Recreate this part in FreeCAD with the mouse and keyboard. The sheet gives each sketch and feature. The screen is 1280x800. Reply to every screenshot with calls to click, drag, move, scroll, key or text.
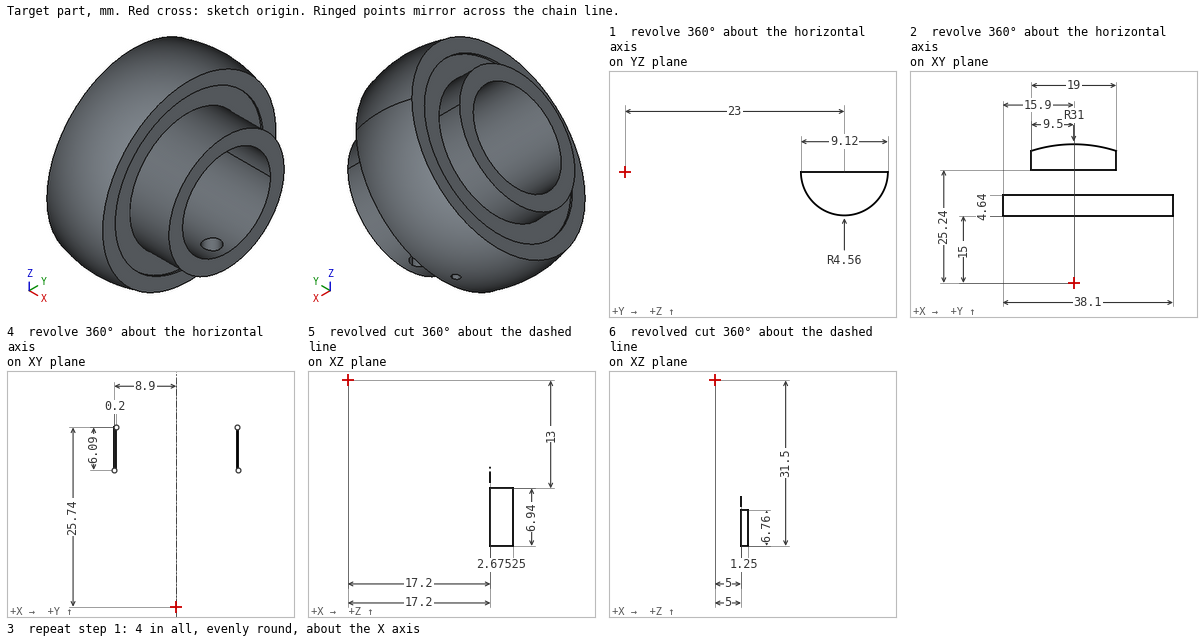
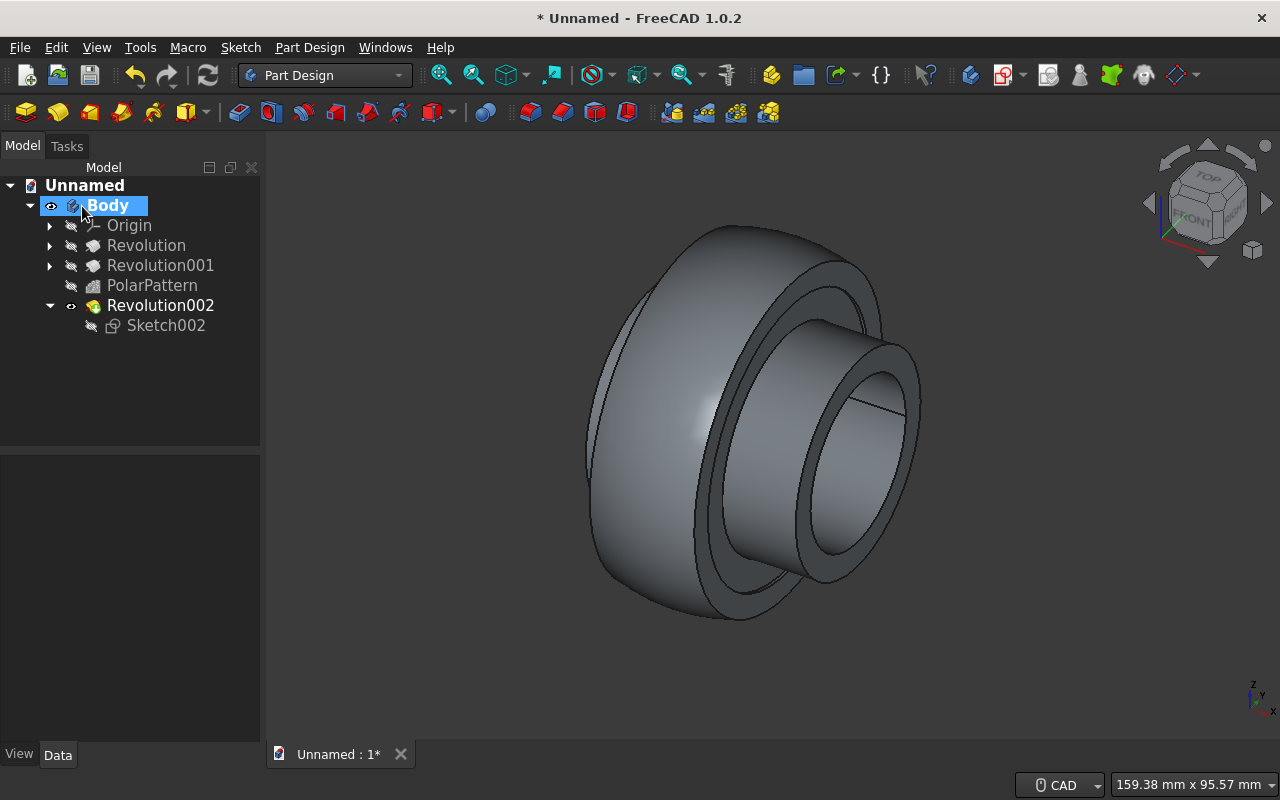
click(1004, 76)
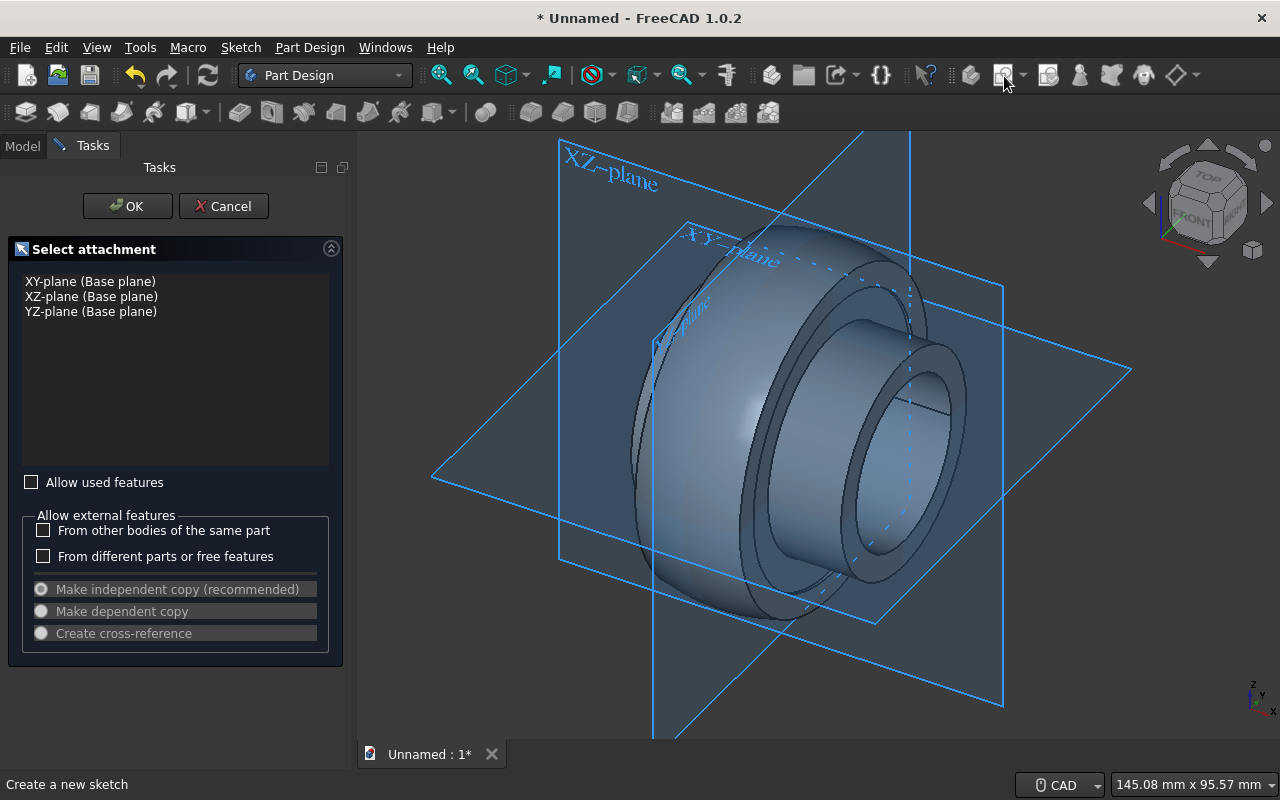
click(82, 296)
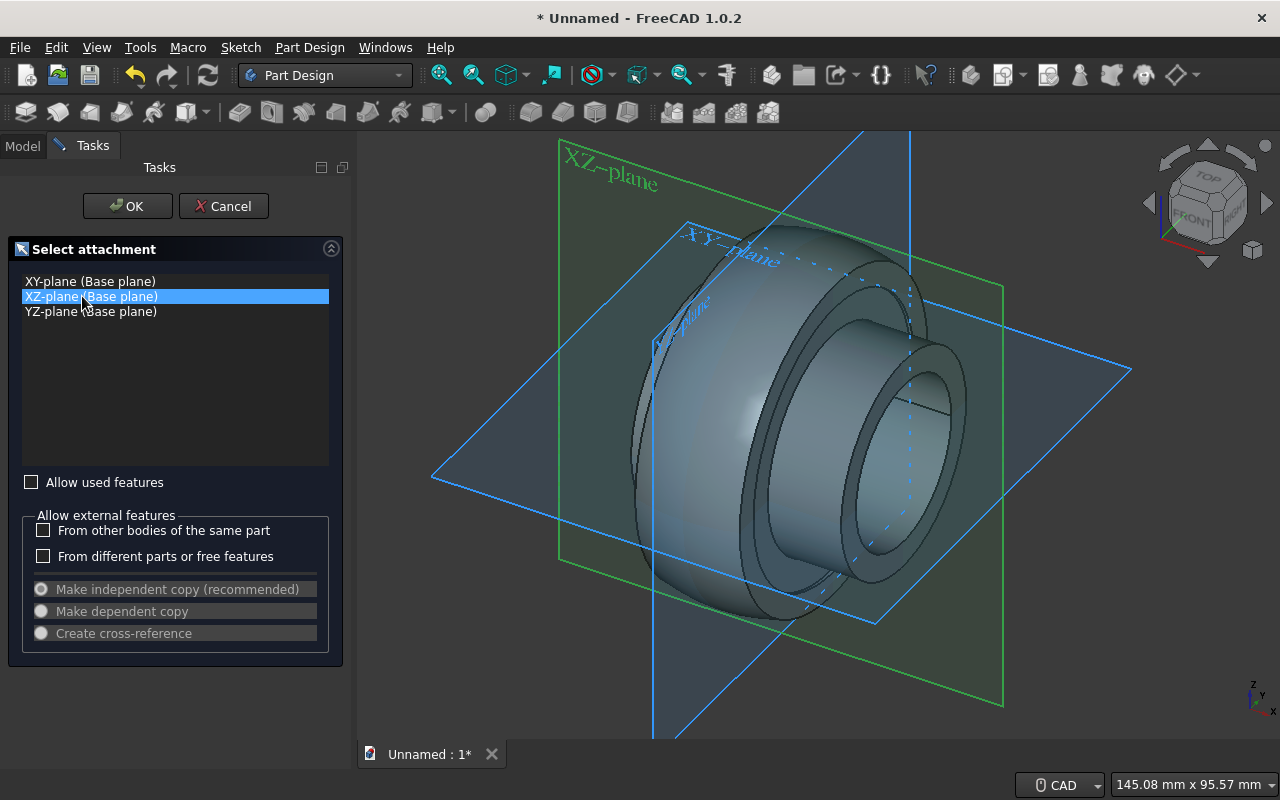
click(128, 206)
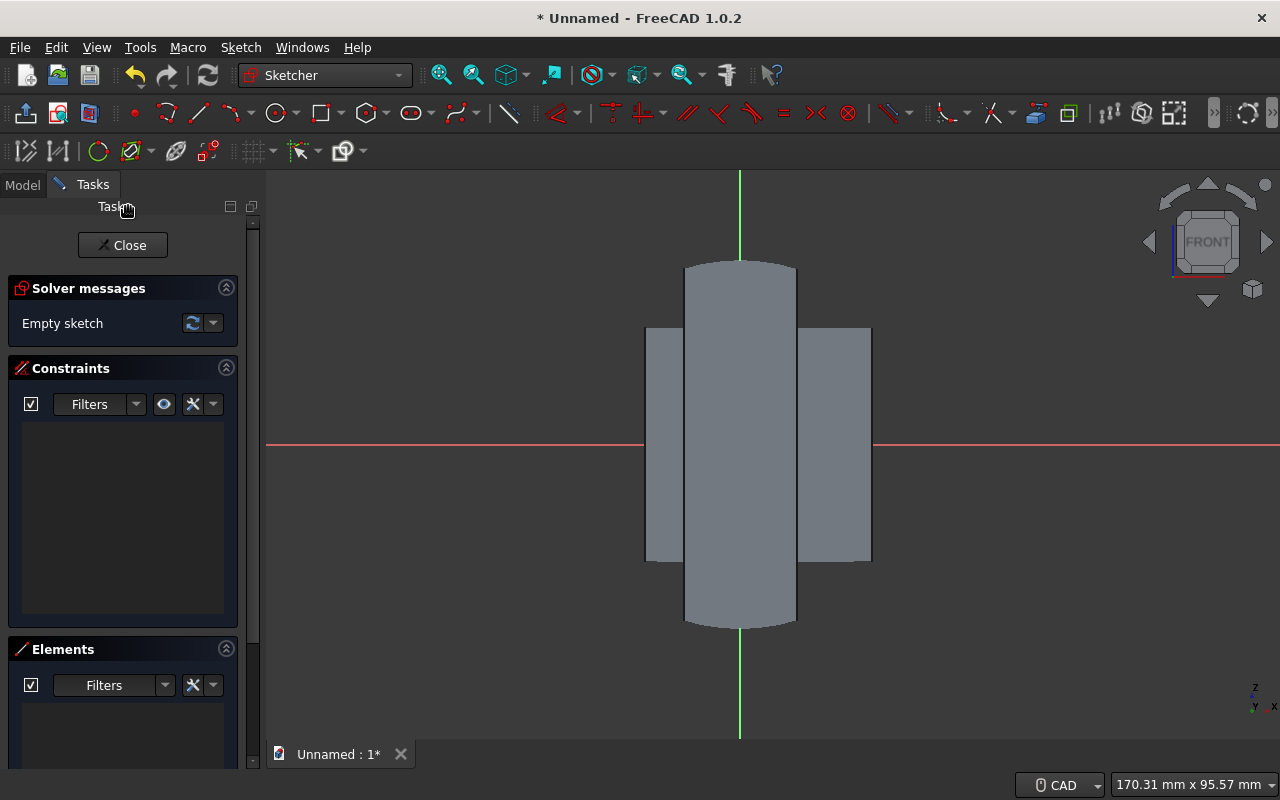
click(90, 114)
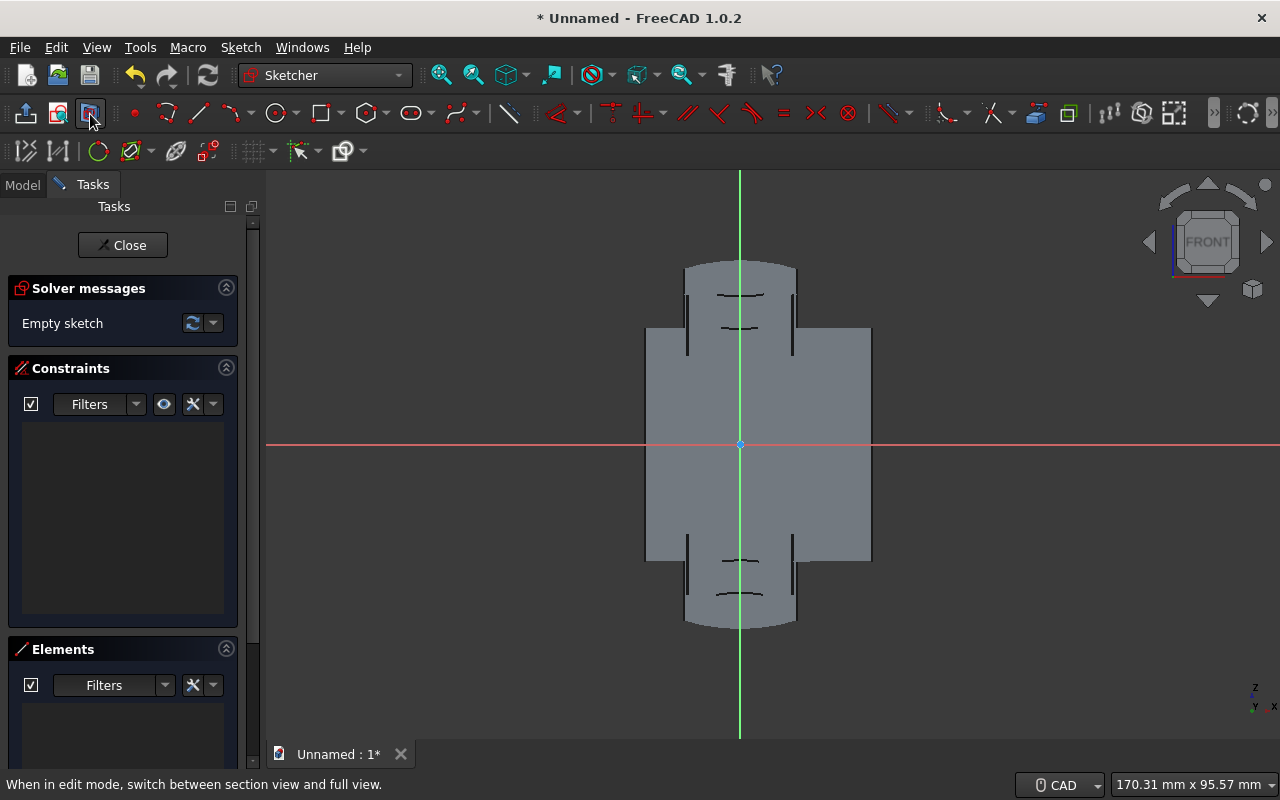
scroll(840, 525, up, 6)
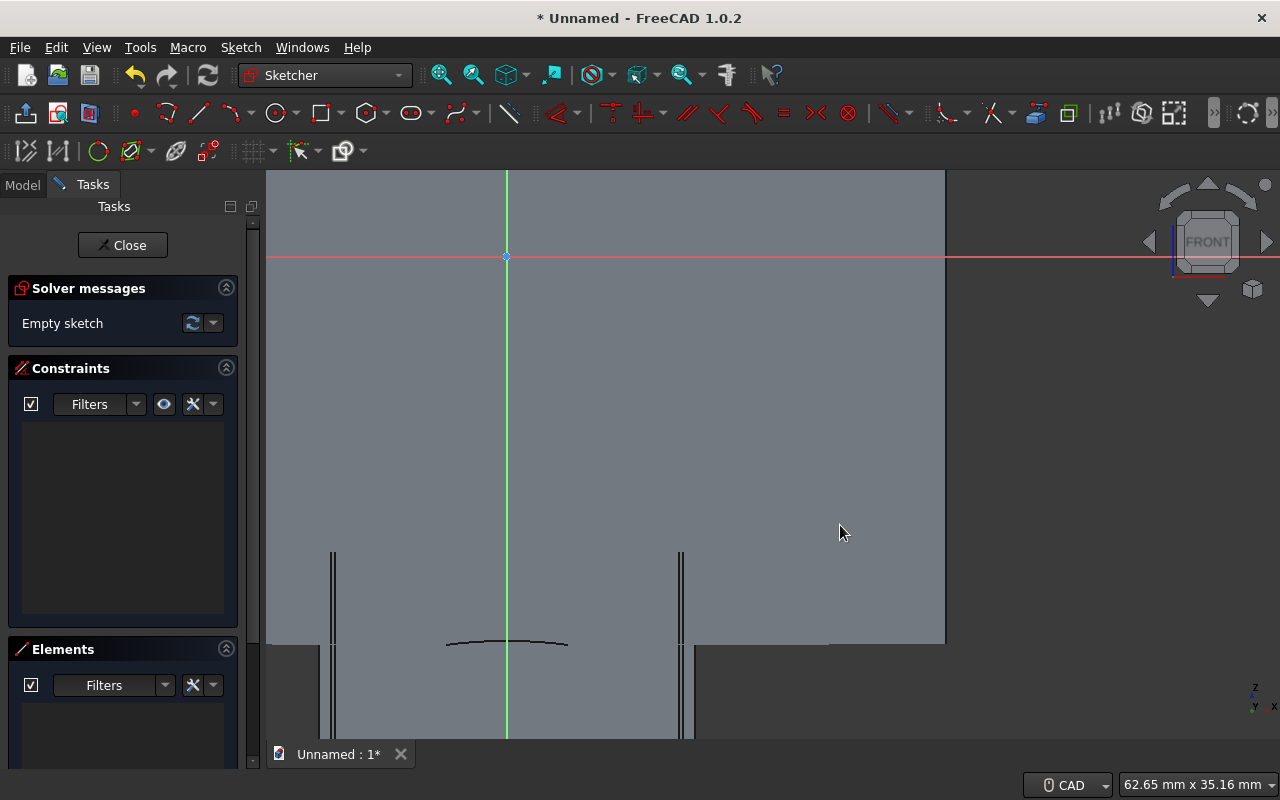
click(322, 114)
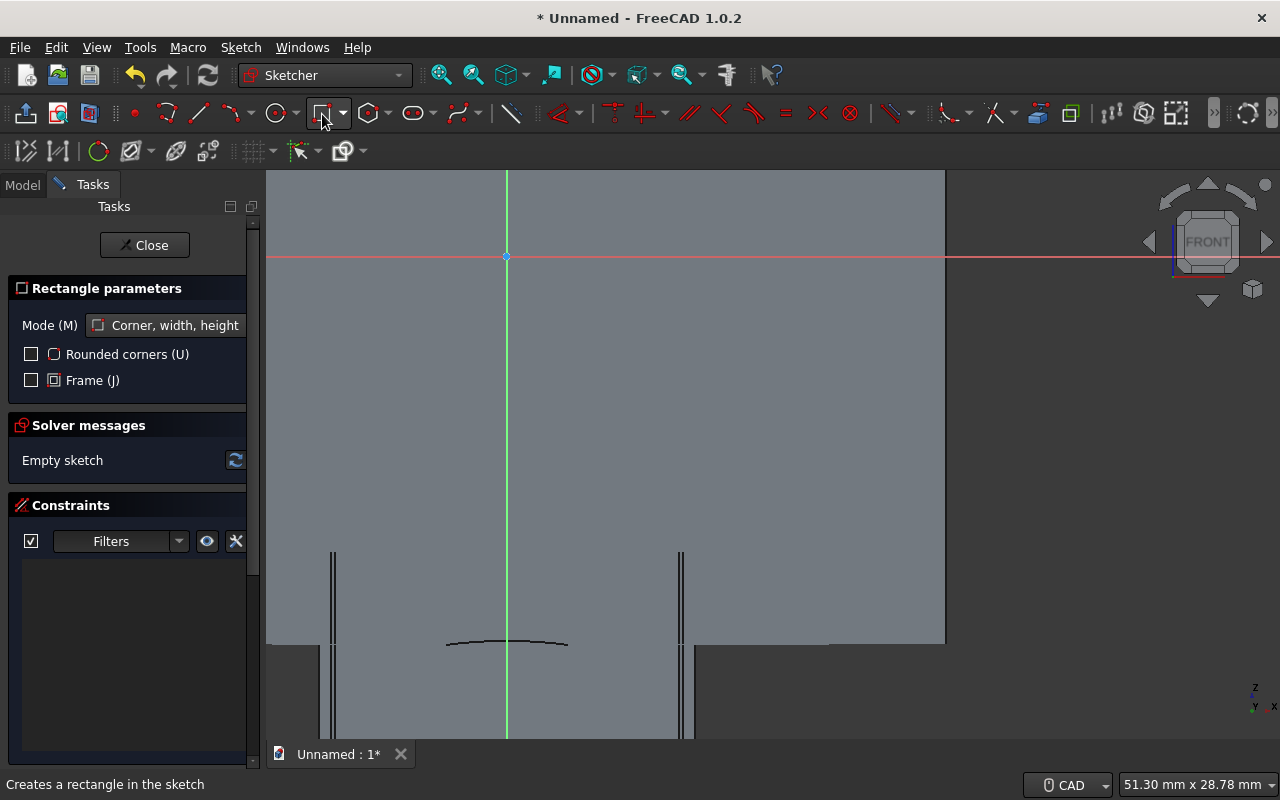
click(847, 514)
click(900, 651)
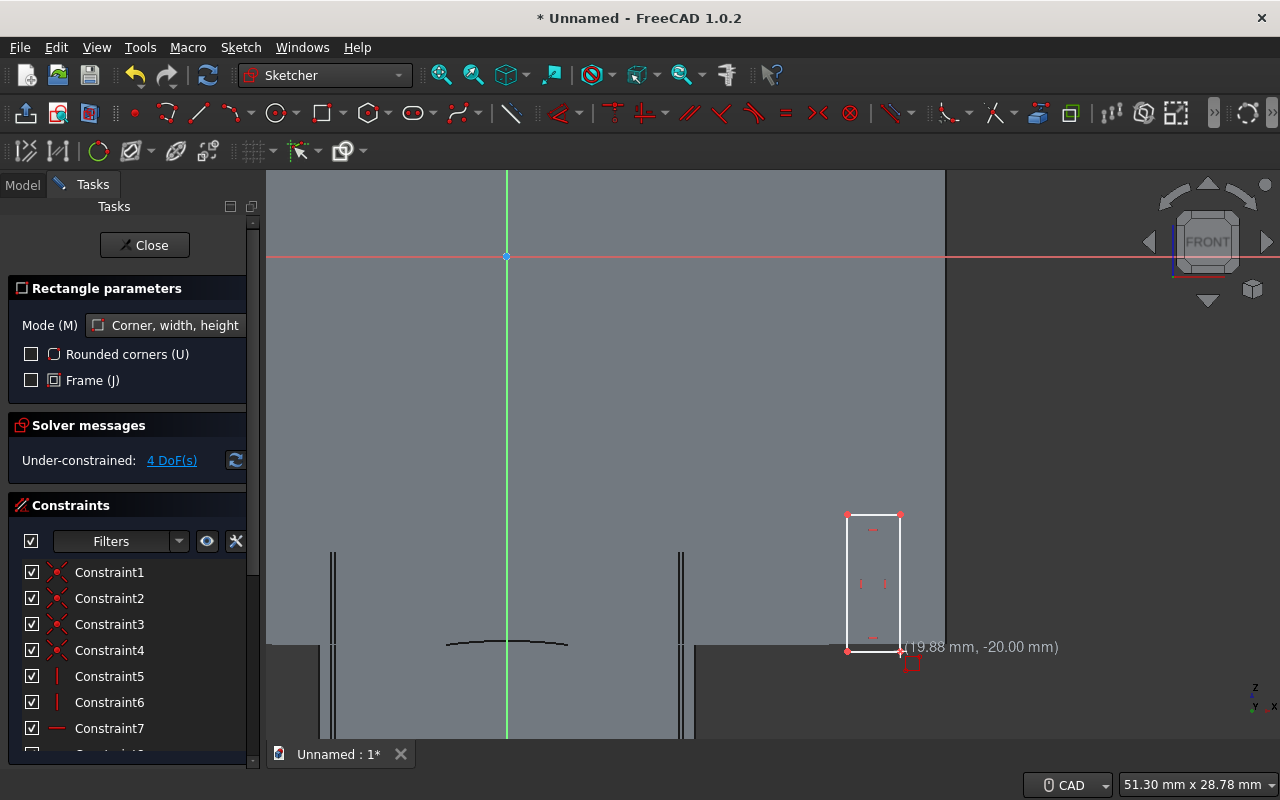
click(200, 114)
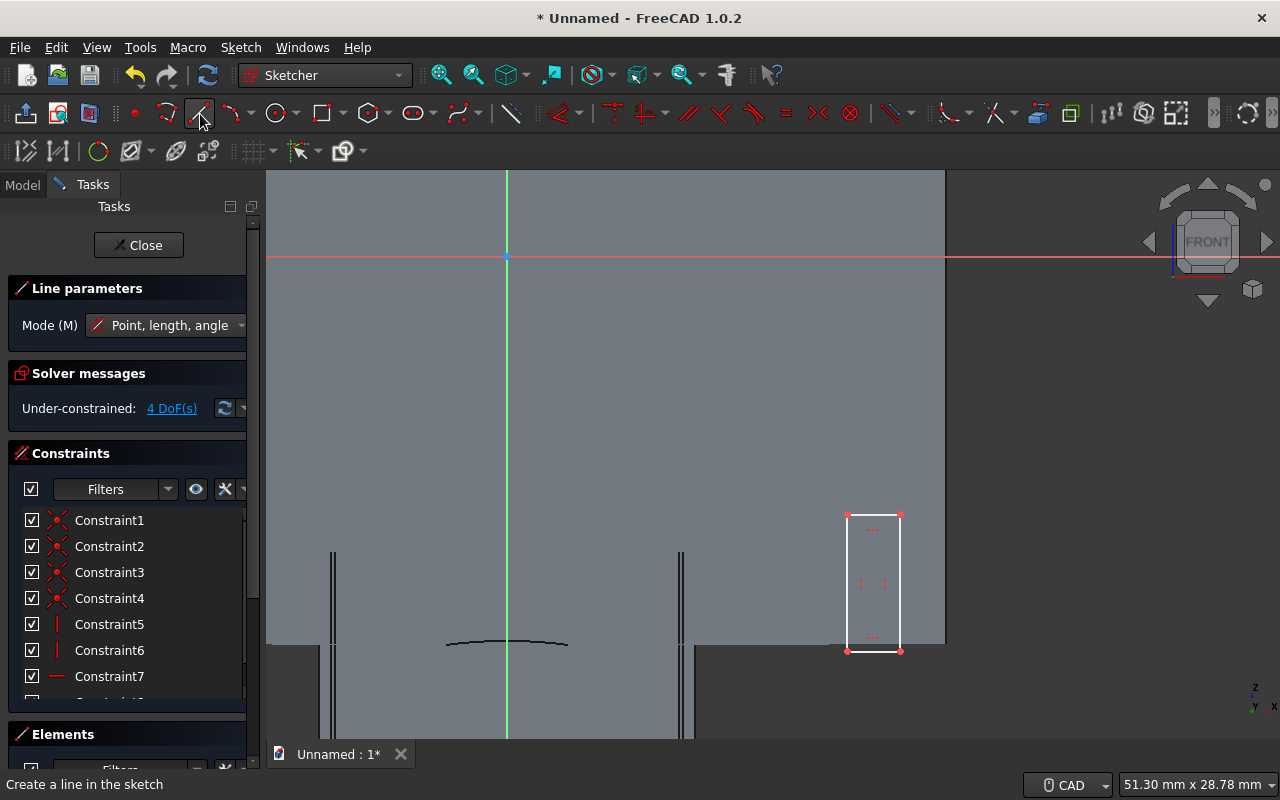
click(847, 500)
click(847, 459)
key(Escape)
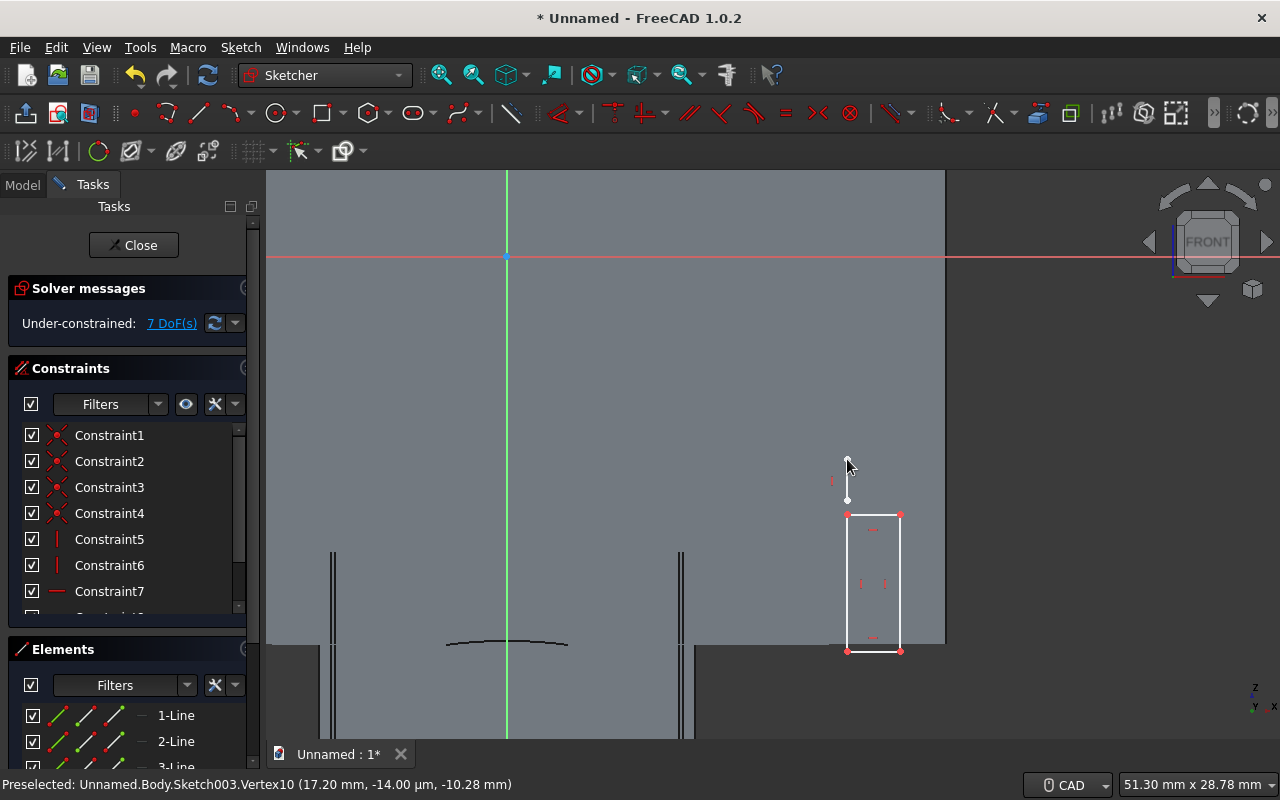
click(847, 489)